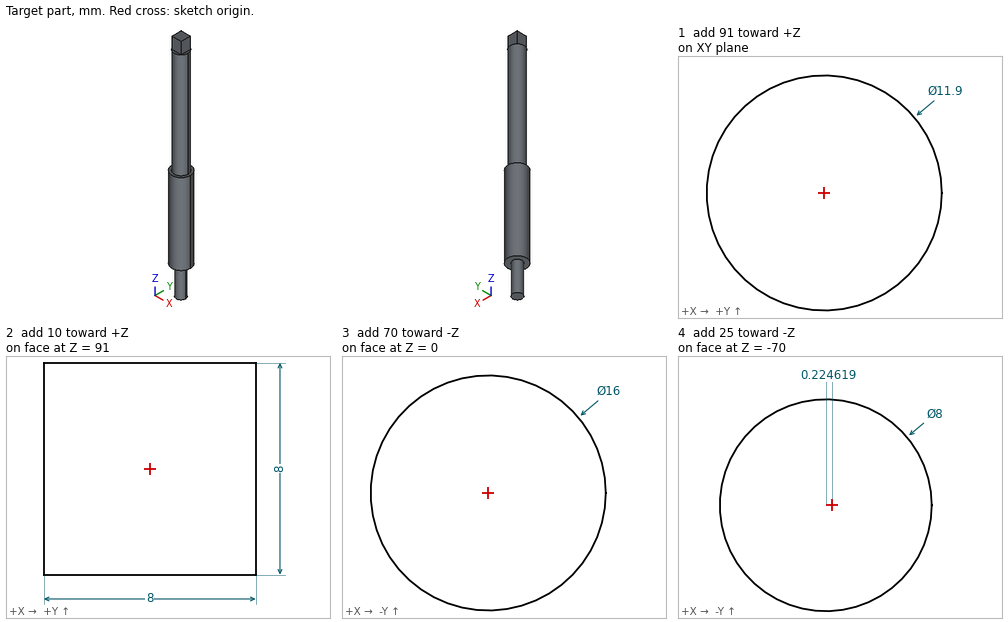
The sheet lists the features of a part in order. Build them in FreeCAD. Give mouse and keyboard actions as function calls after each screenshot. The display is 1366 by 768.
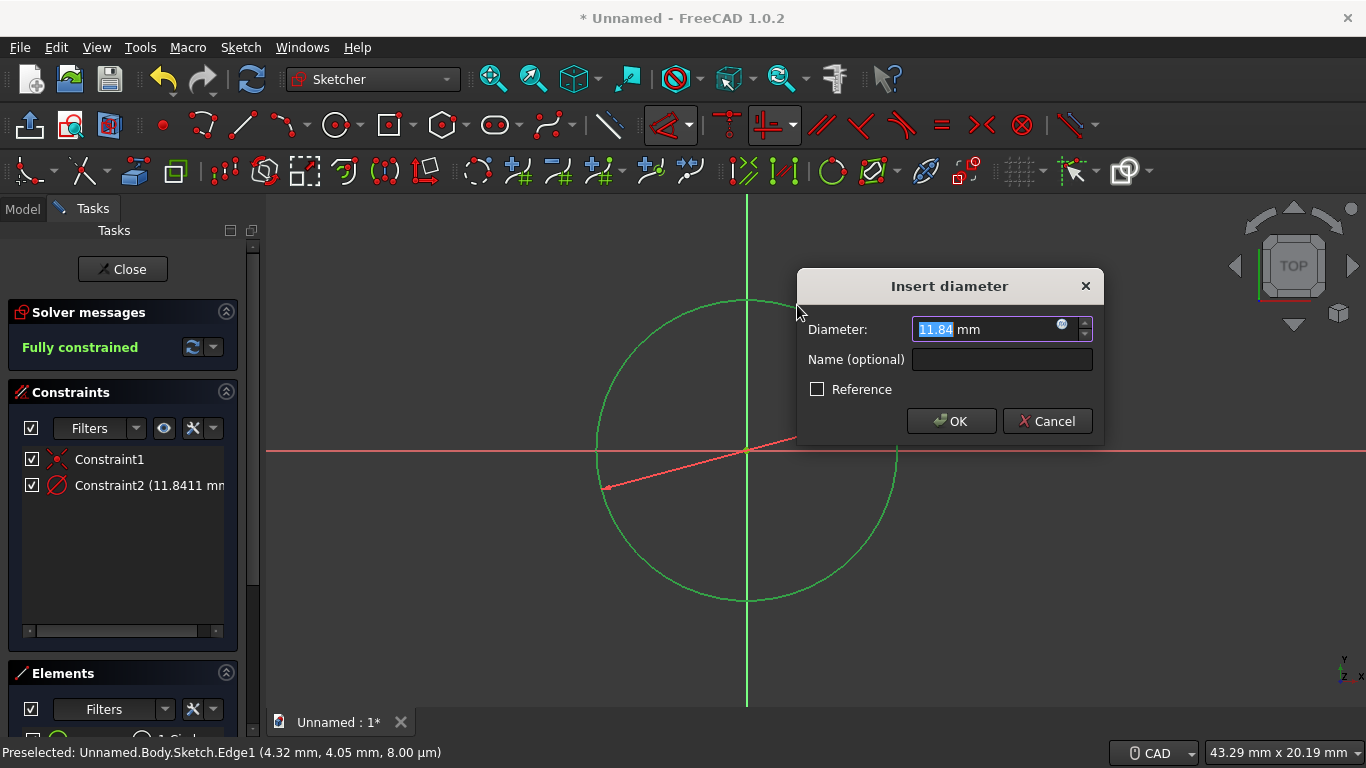
text(11.9)
key(Return)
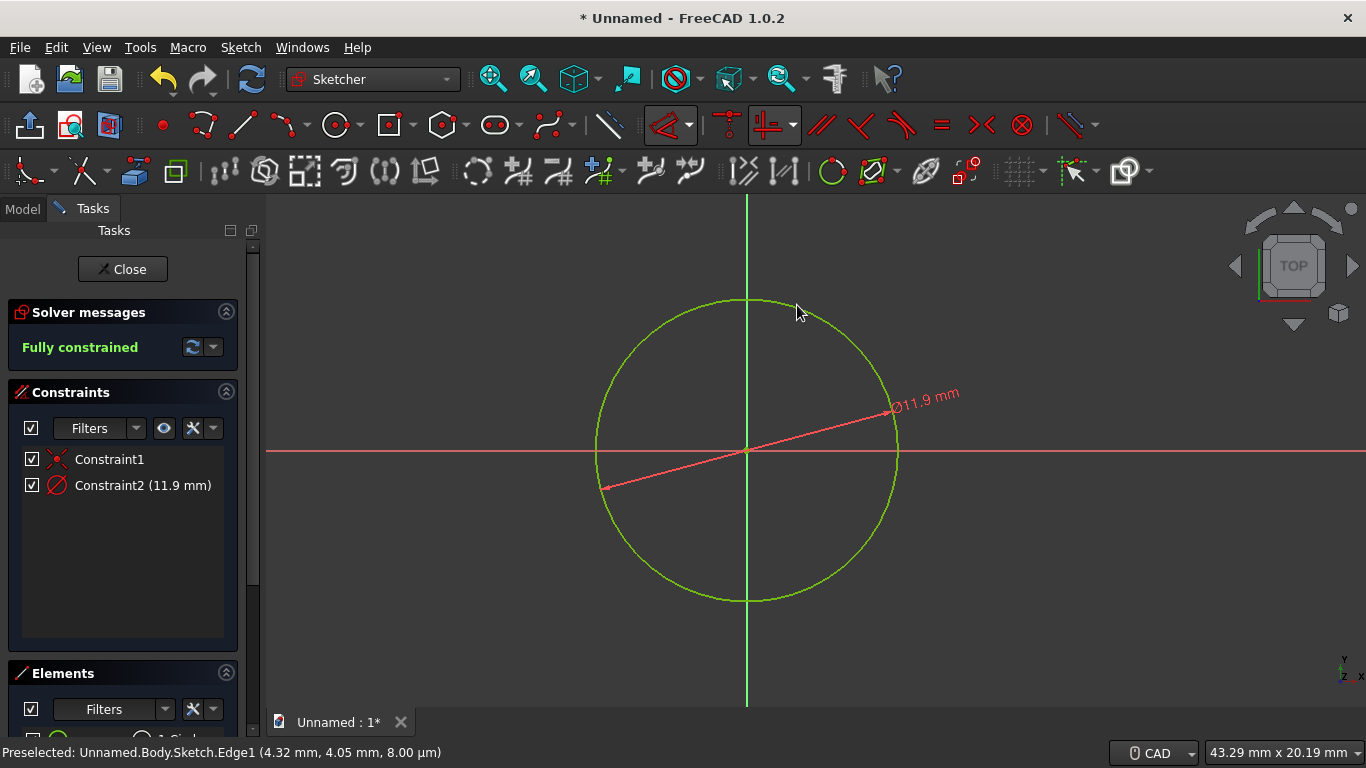
click(123, 269)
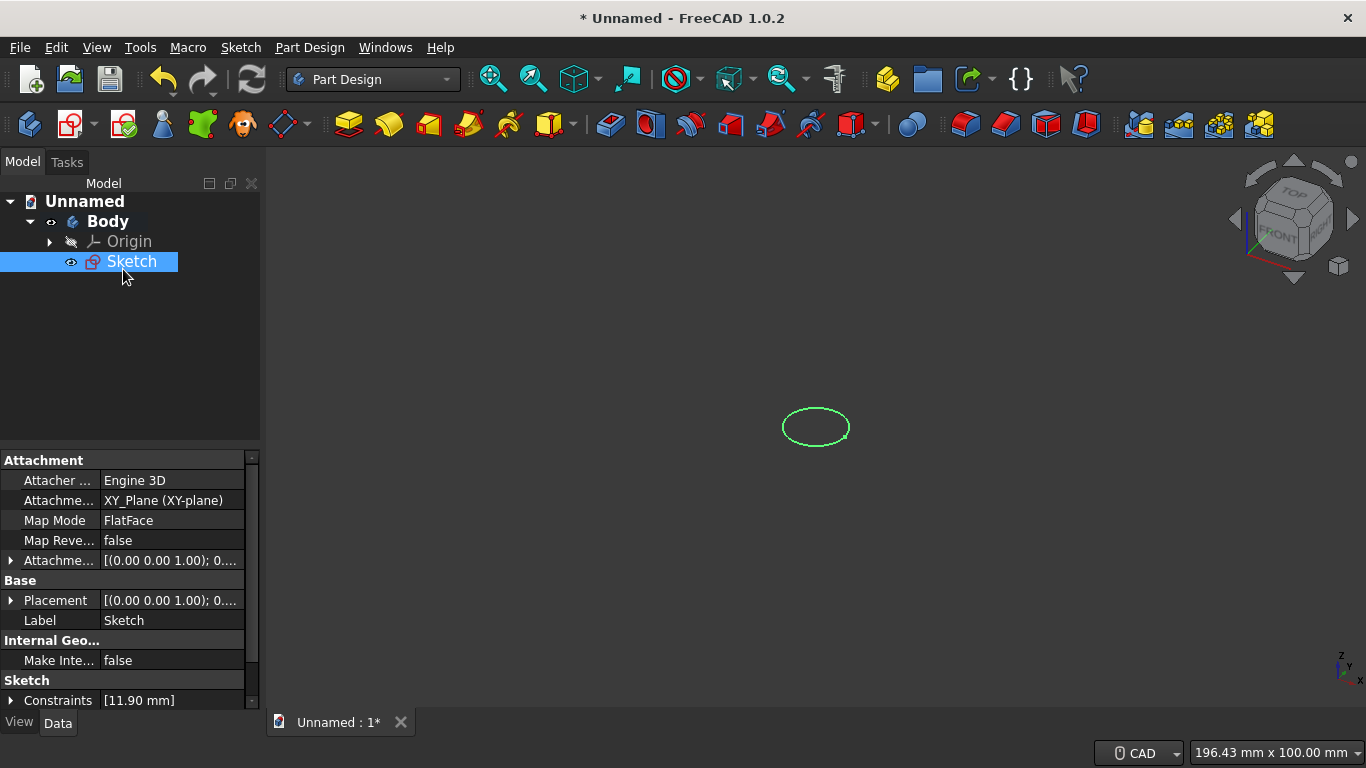
click(350, 124)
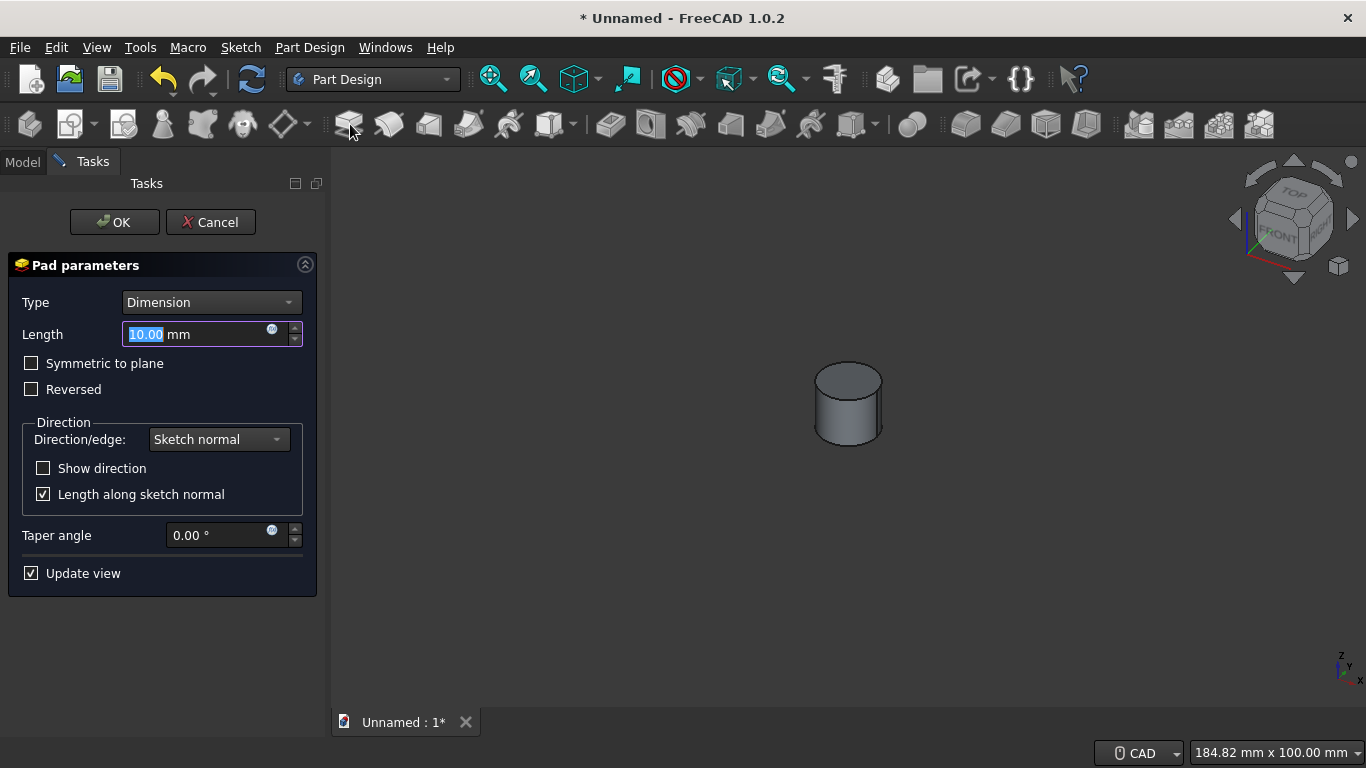
text(91)
key(Tab)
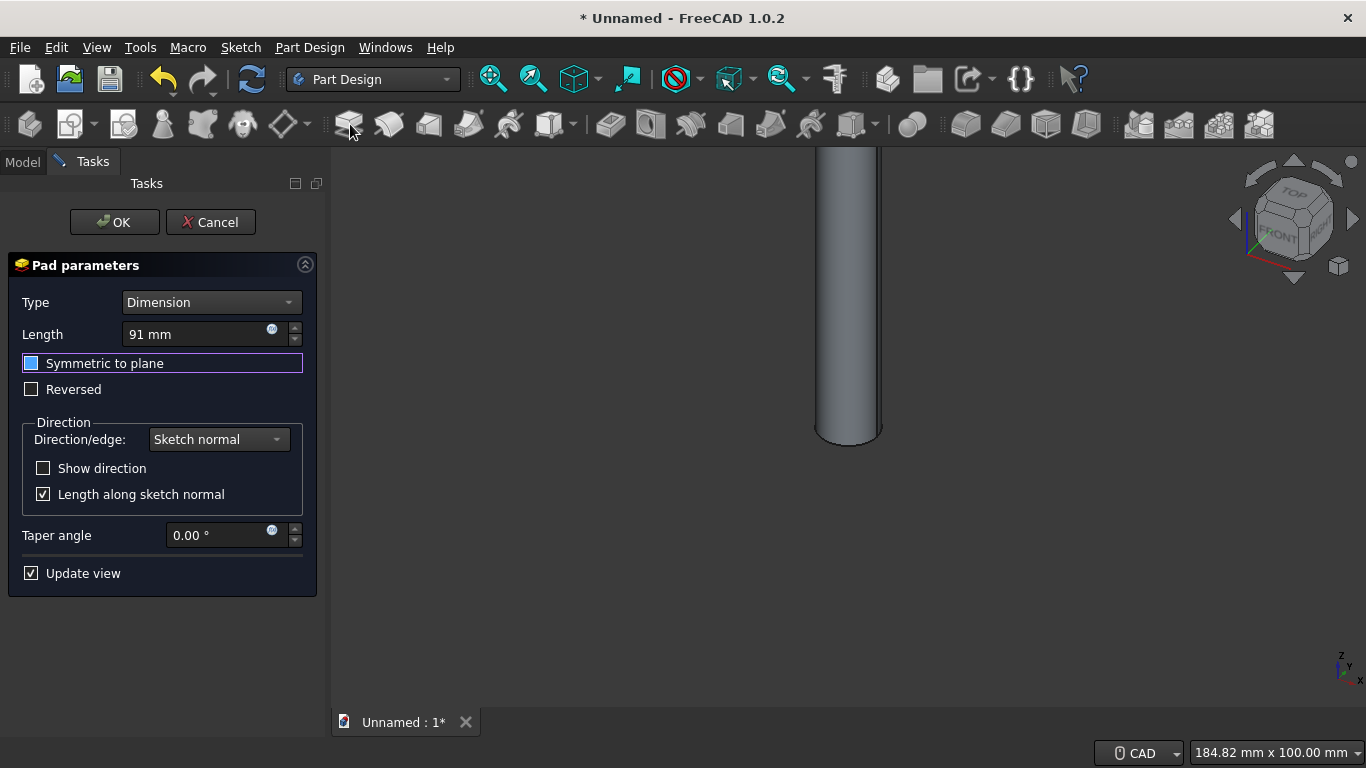
click(115, 222)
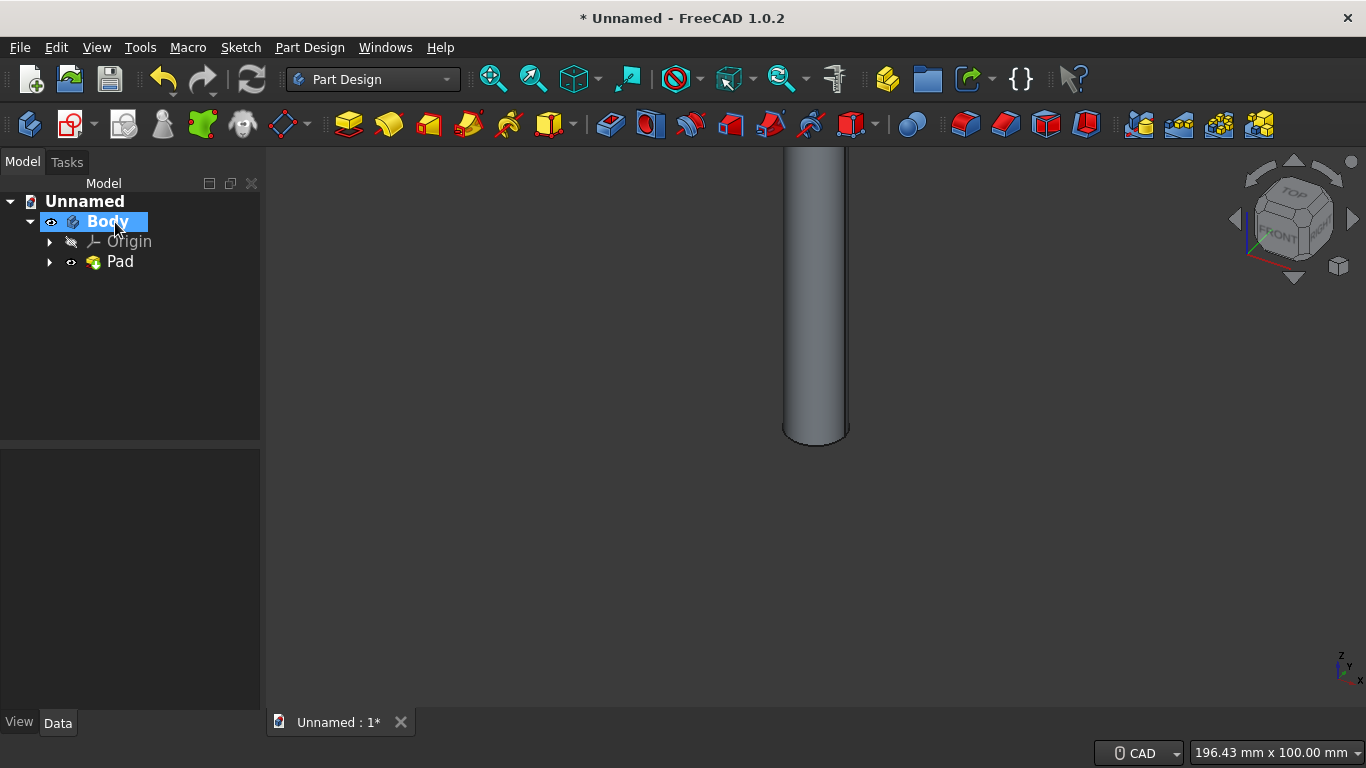
click(494, 80)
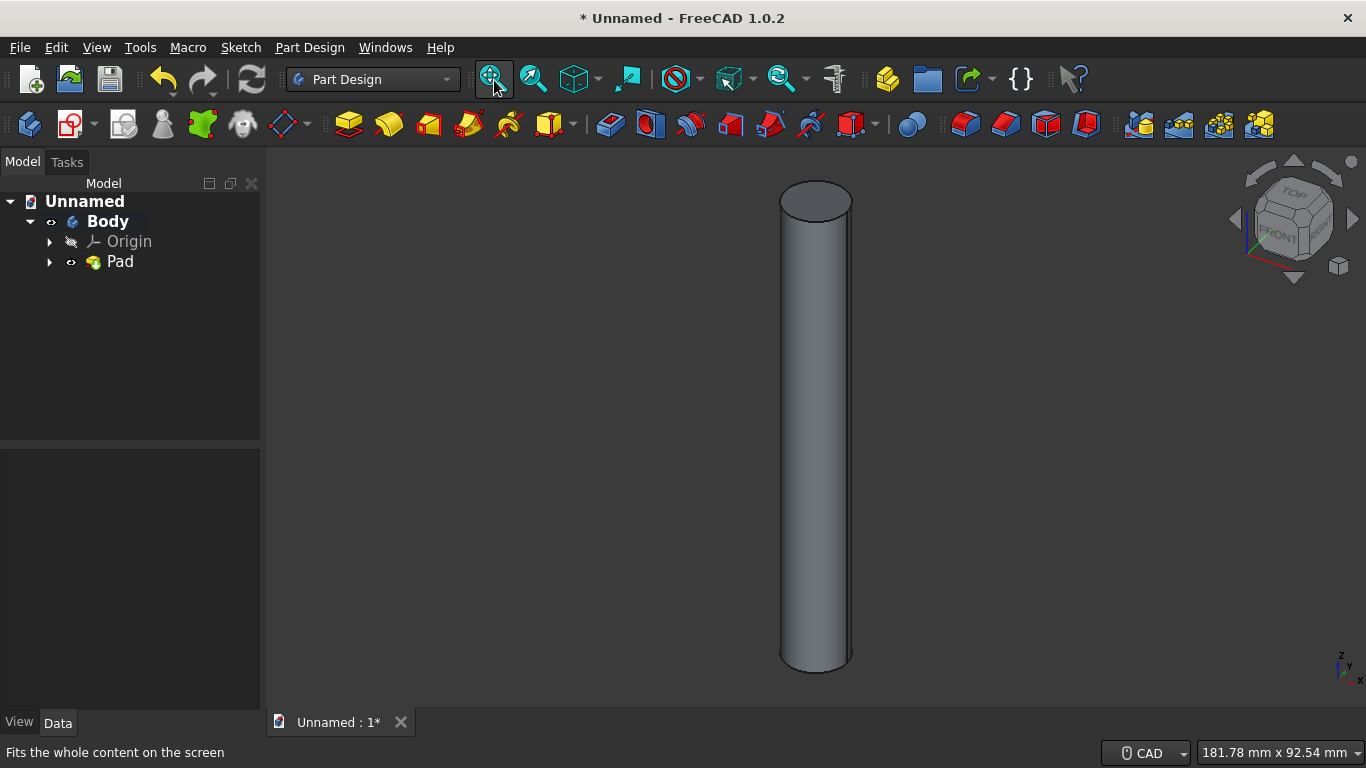
click(816, 200)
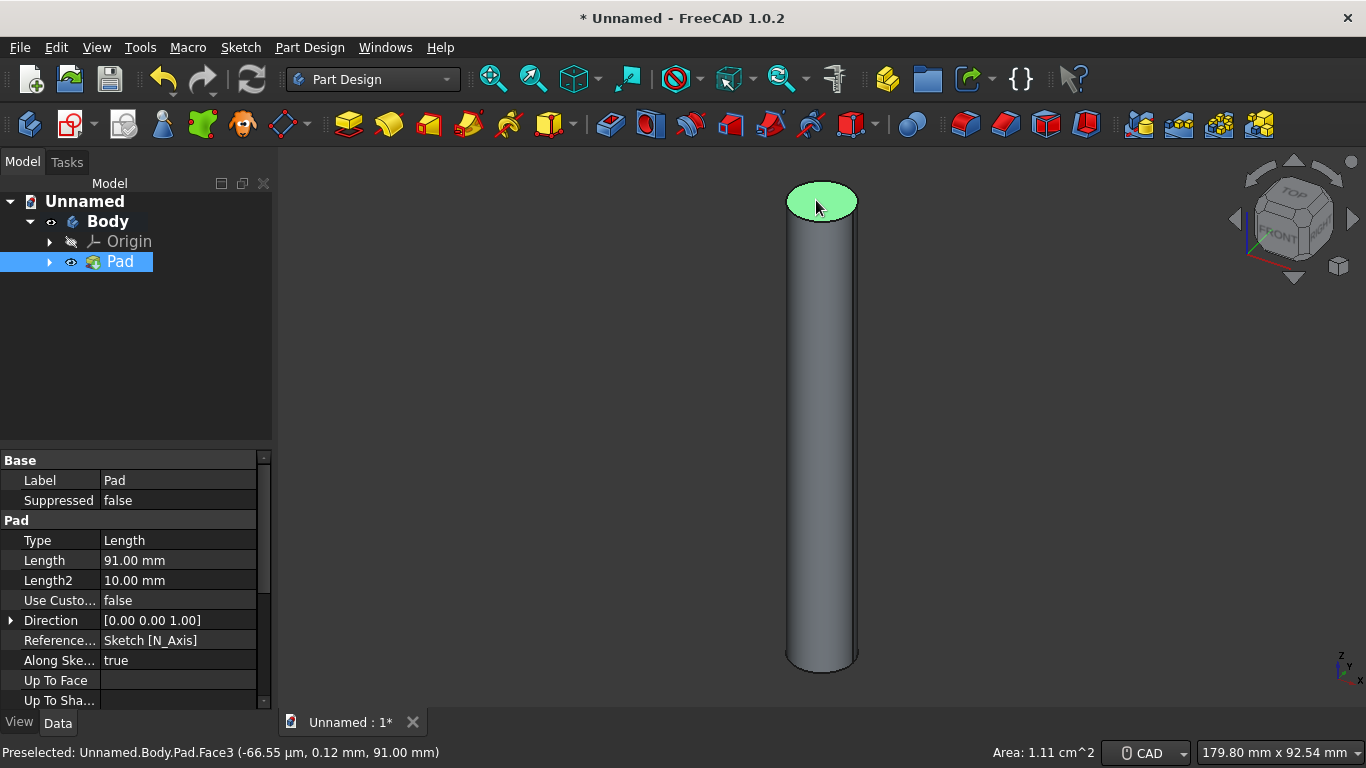
click(70, 124)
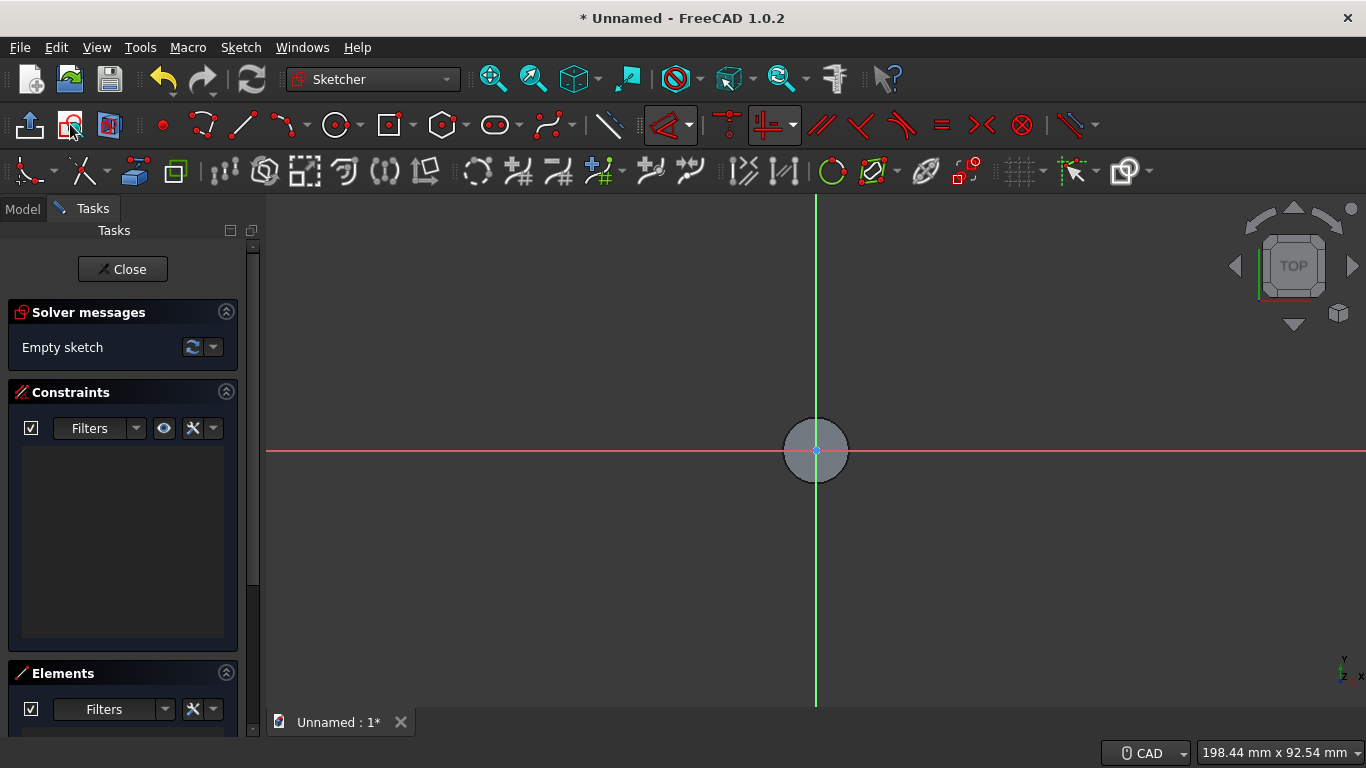
scroll(827, 450, up, 10)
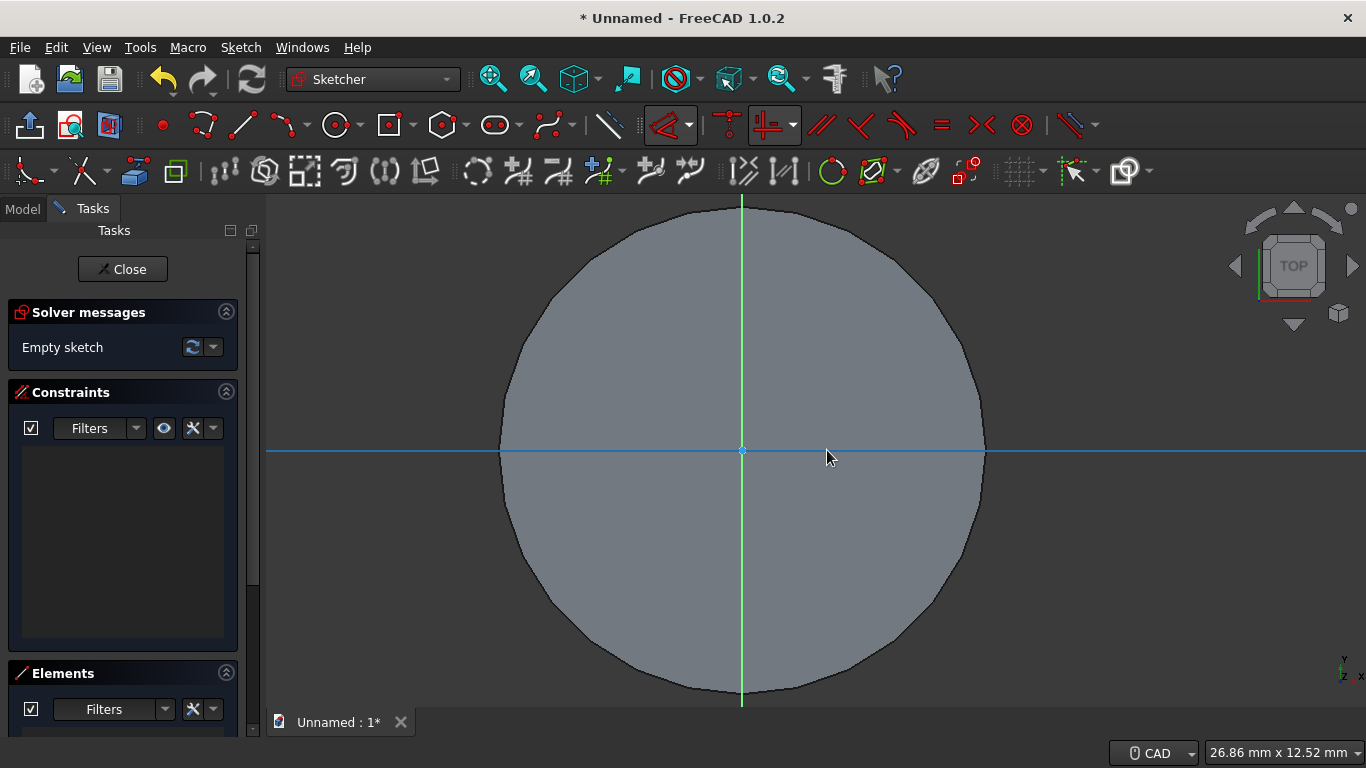
click(390, 126)